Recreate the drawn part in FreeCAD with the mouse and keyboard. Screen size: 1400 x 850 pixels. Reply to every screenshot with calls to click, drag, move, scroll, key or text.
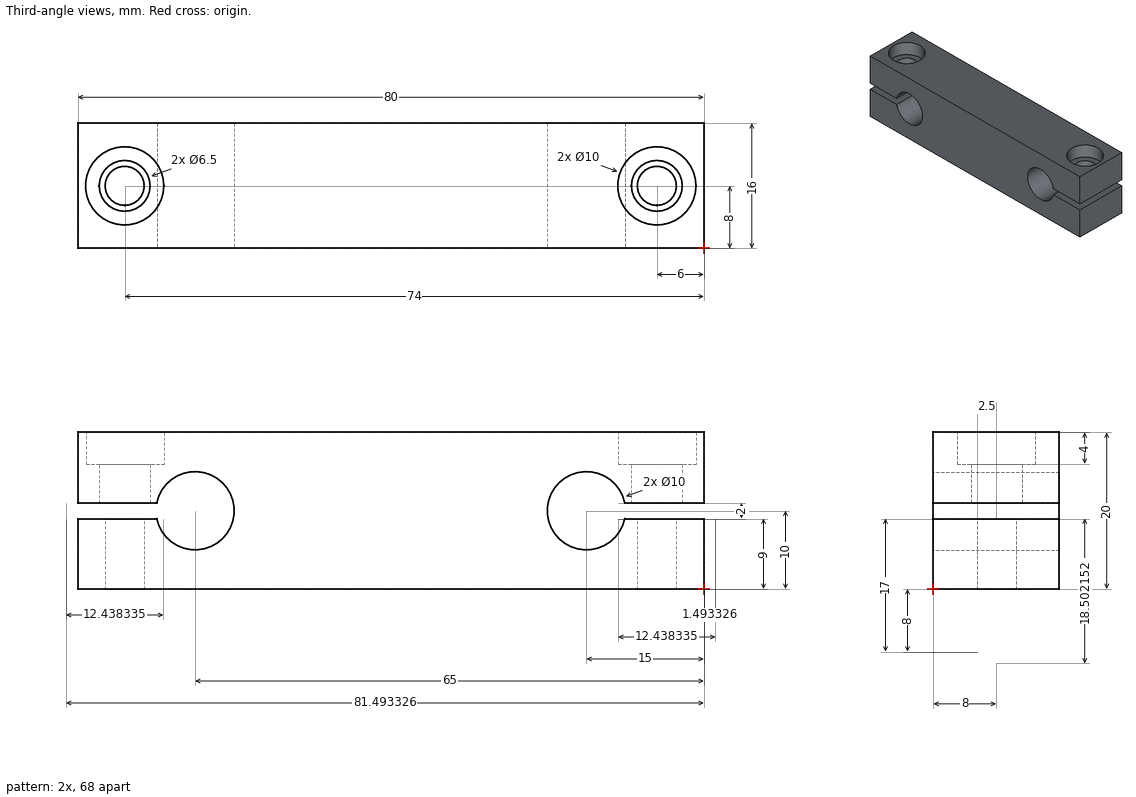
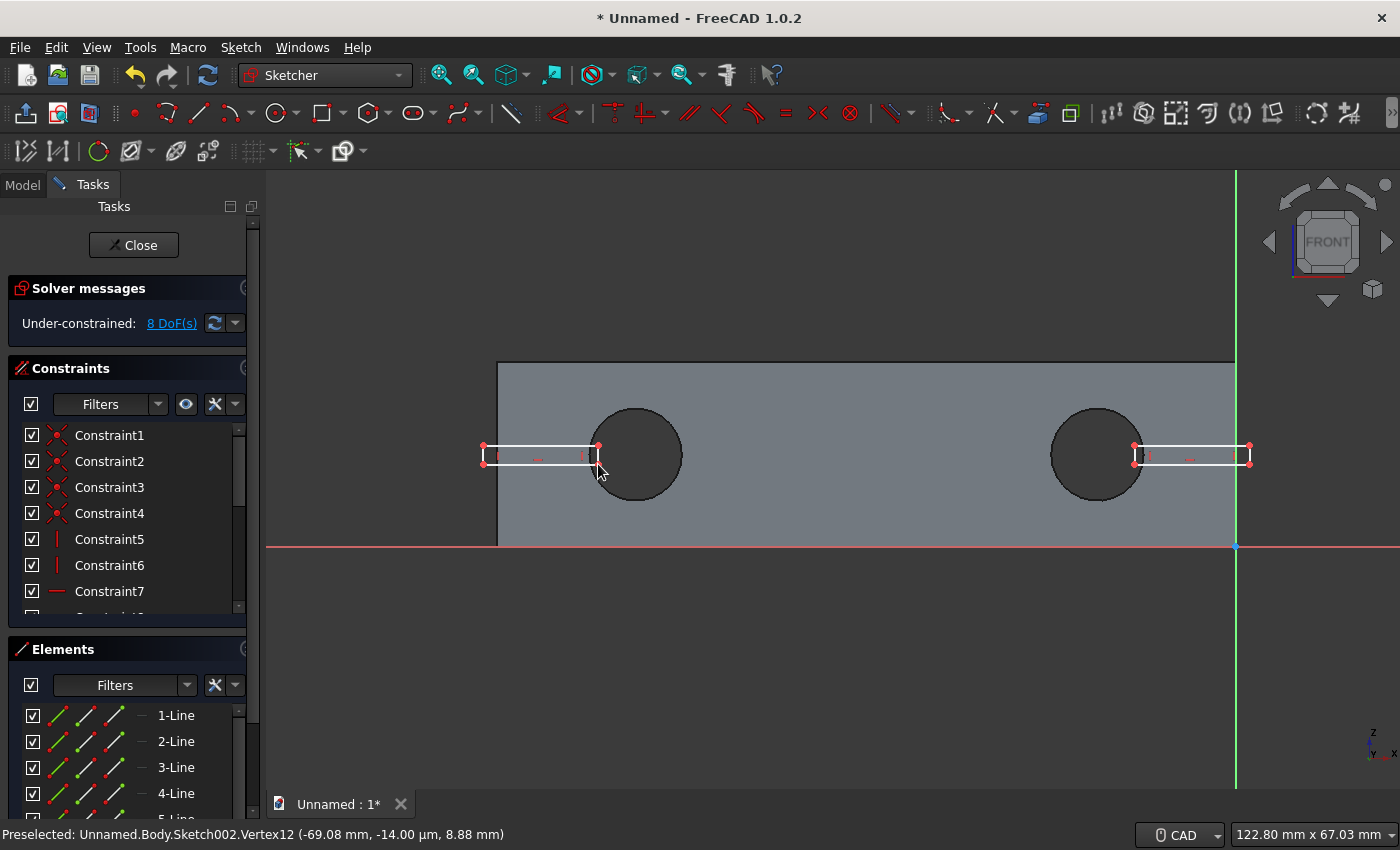
click(558, 114)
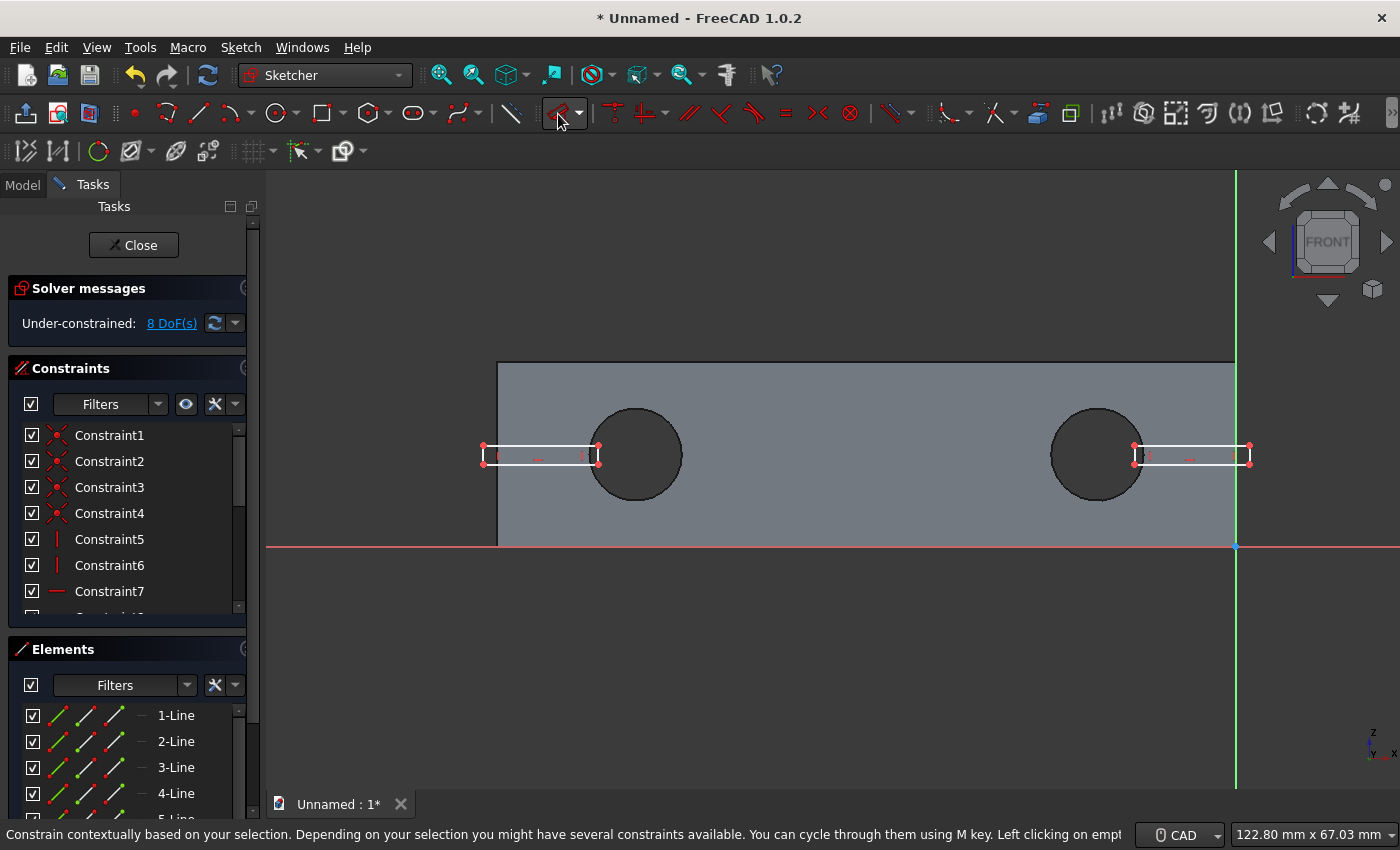
scroll(1135, 455, up, 4)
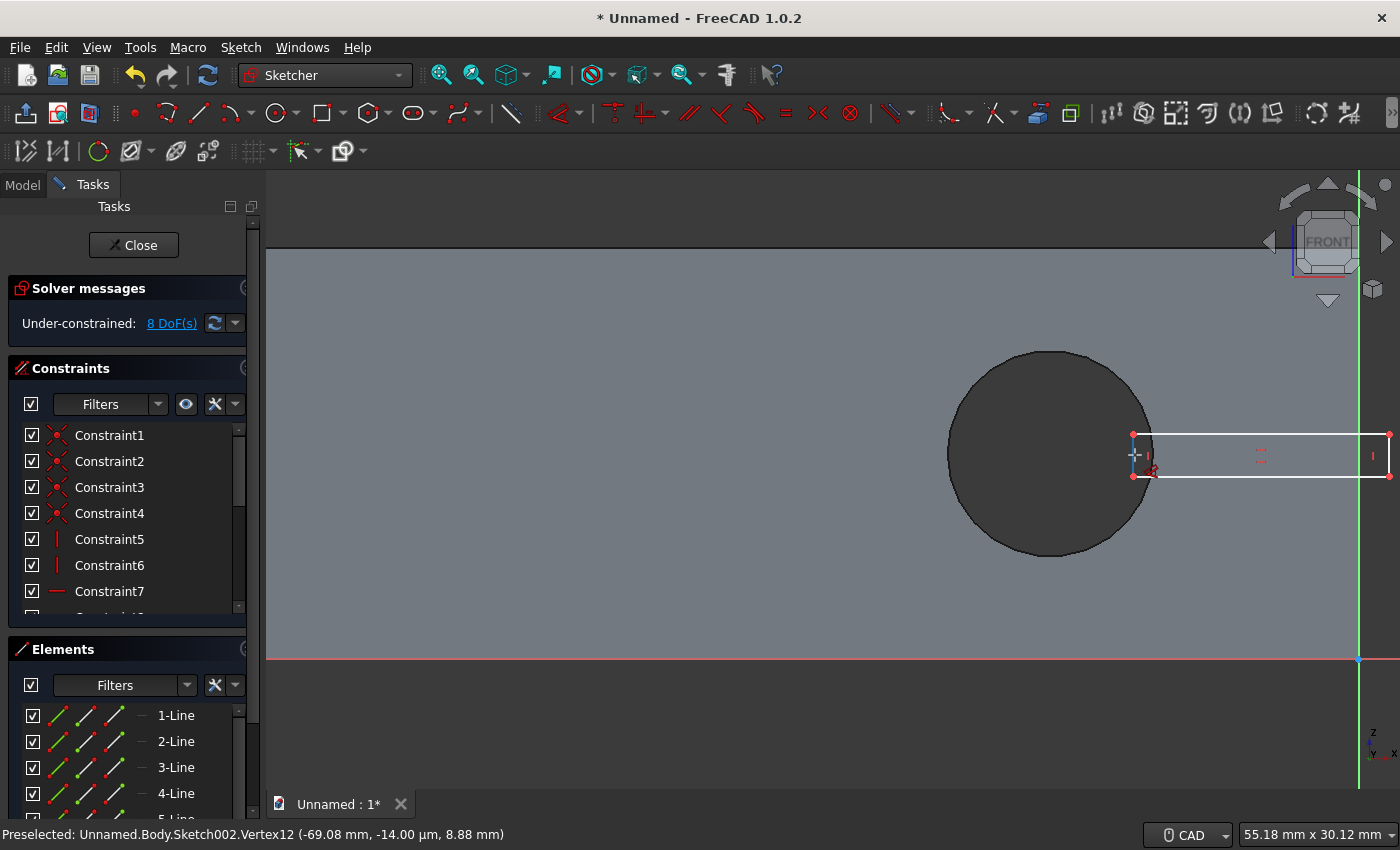
click(1133, 456)
click(1167, 456)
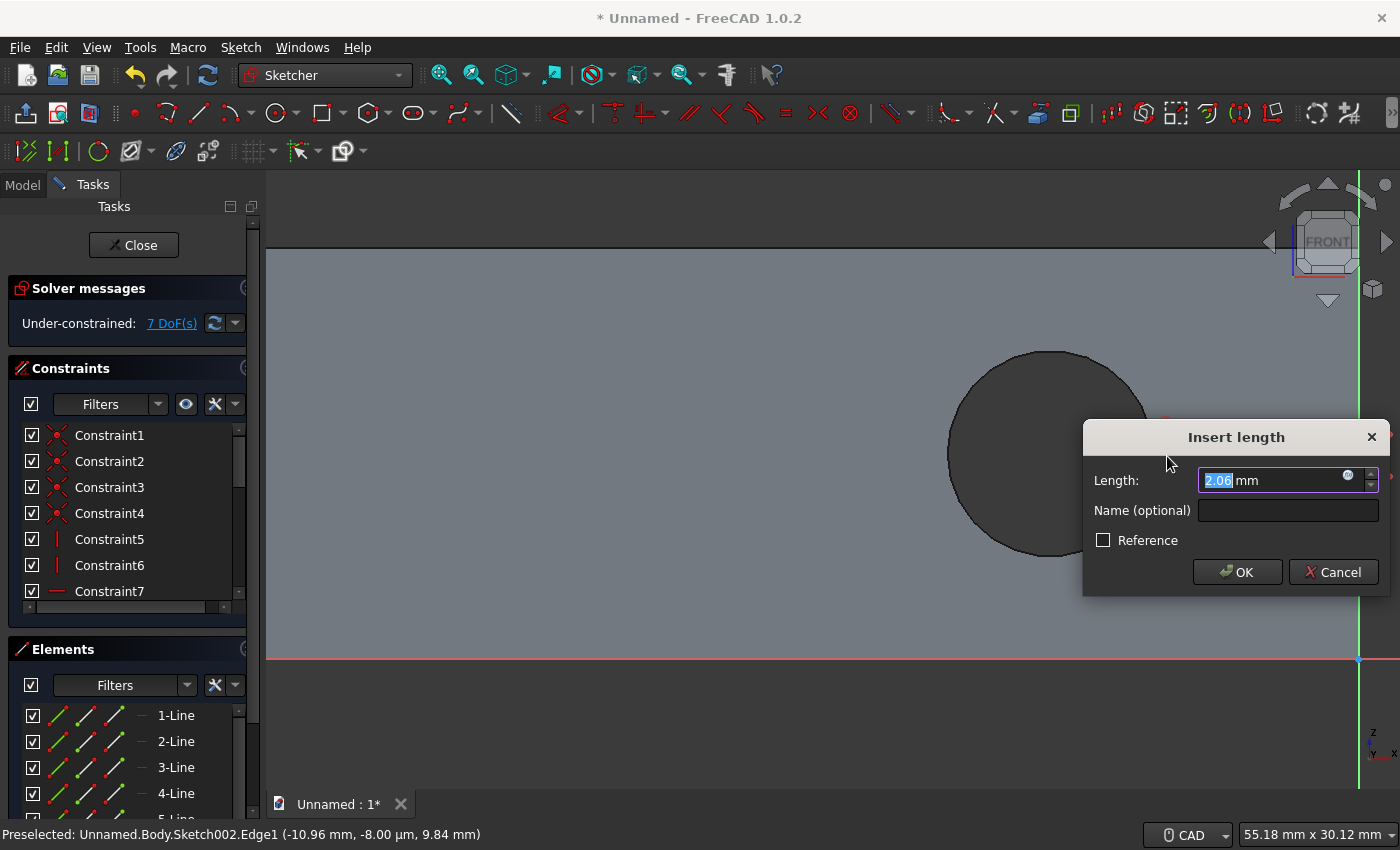
text(2)
key(Return)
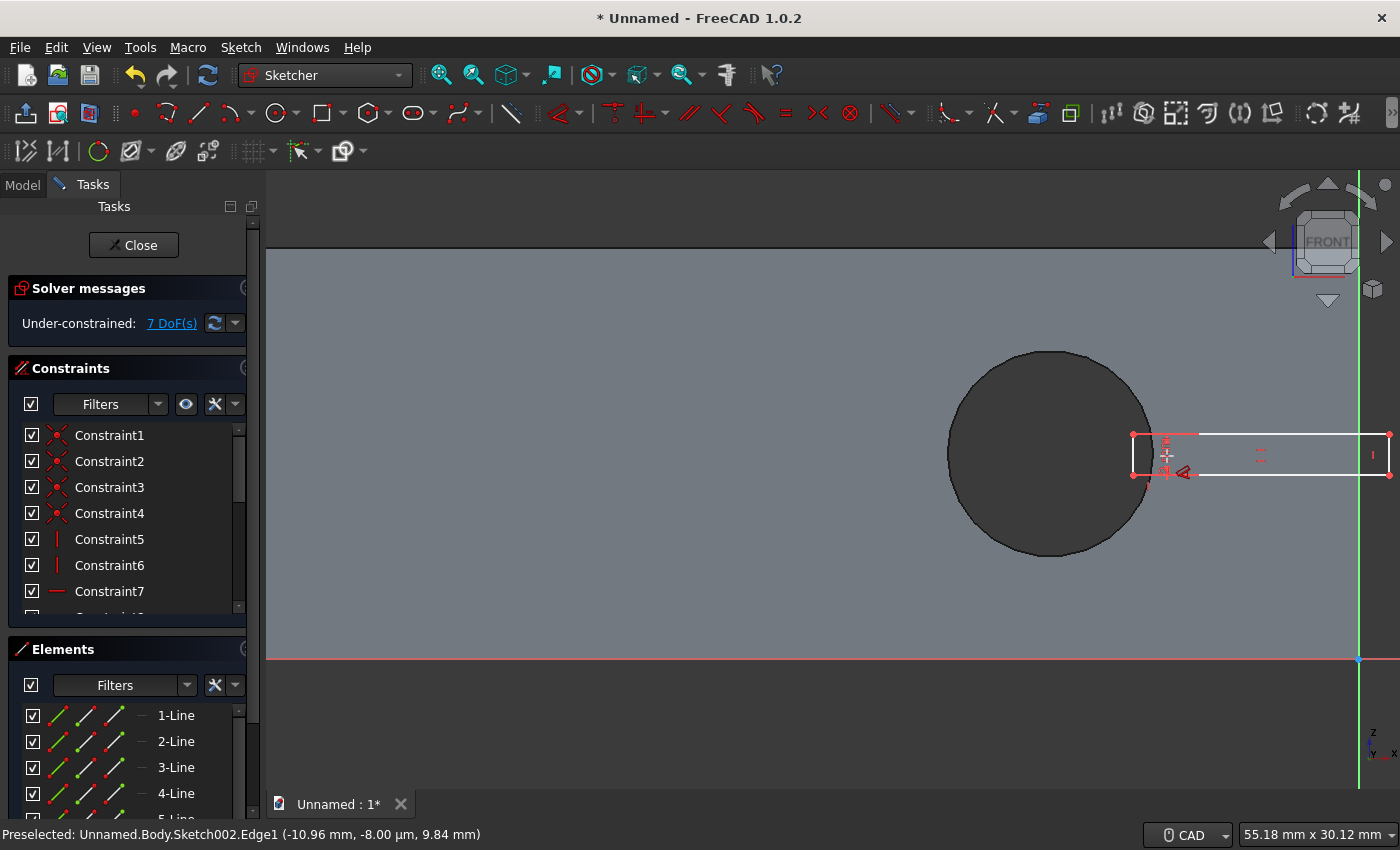
scroll(897, 441, down, 5)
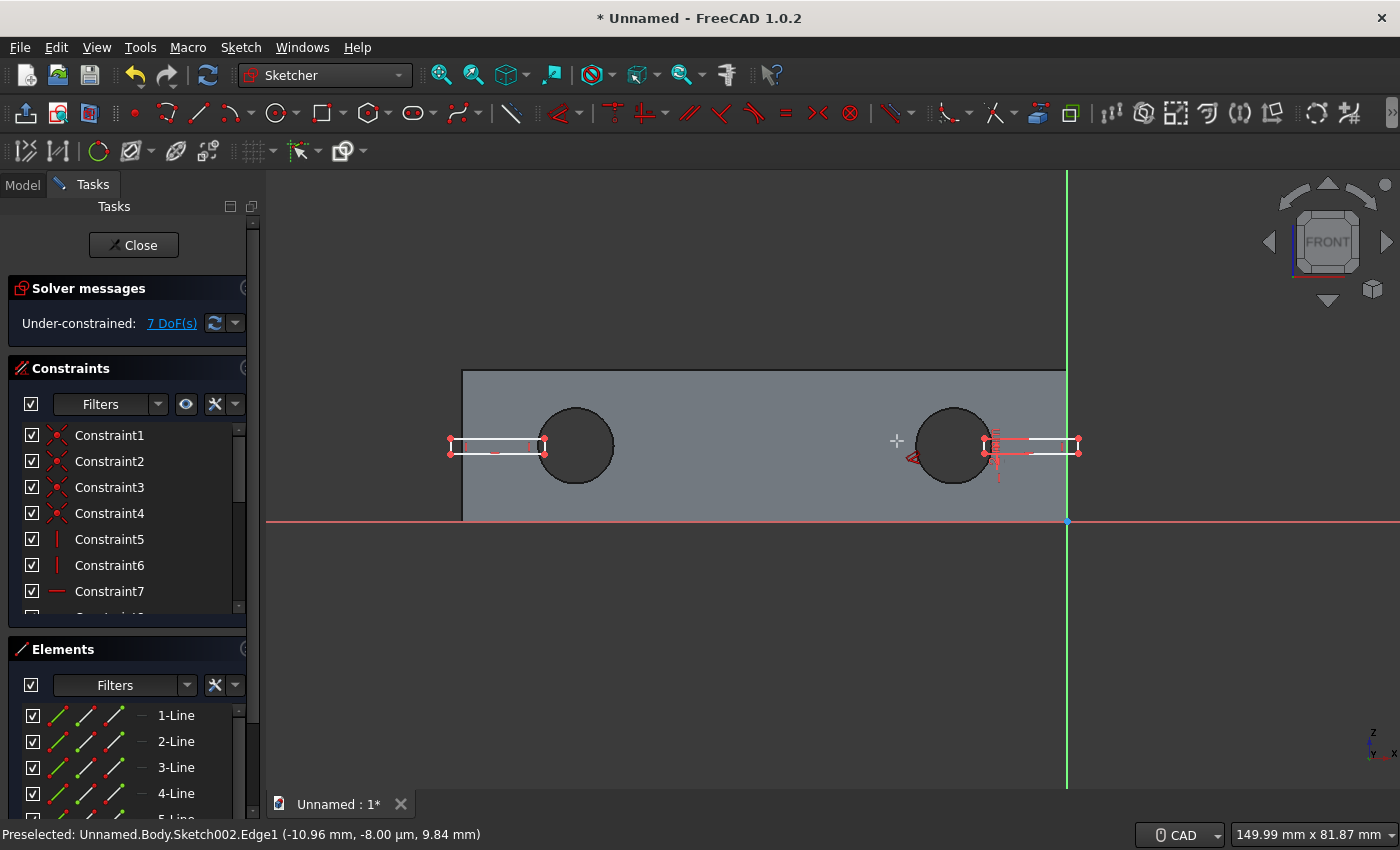
scroll(451, 444, up, 6)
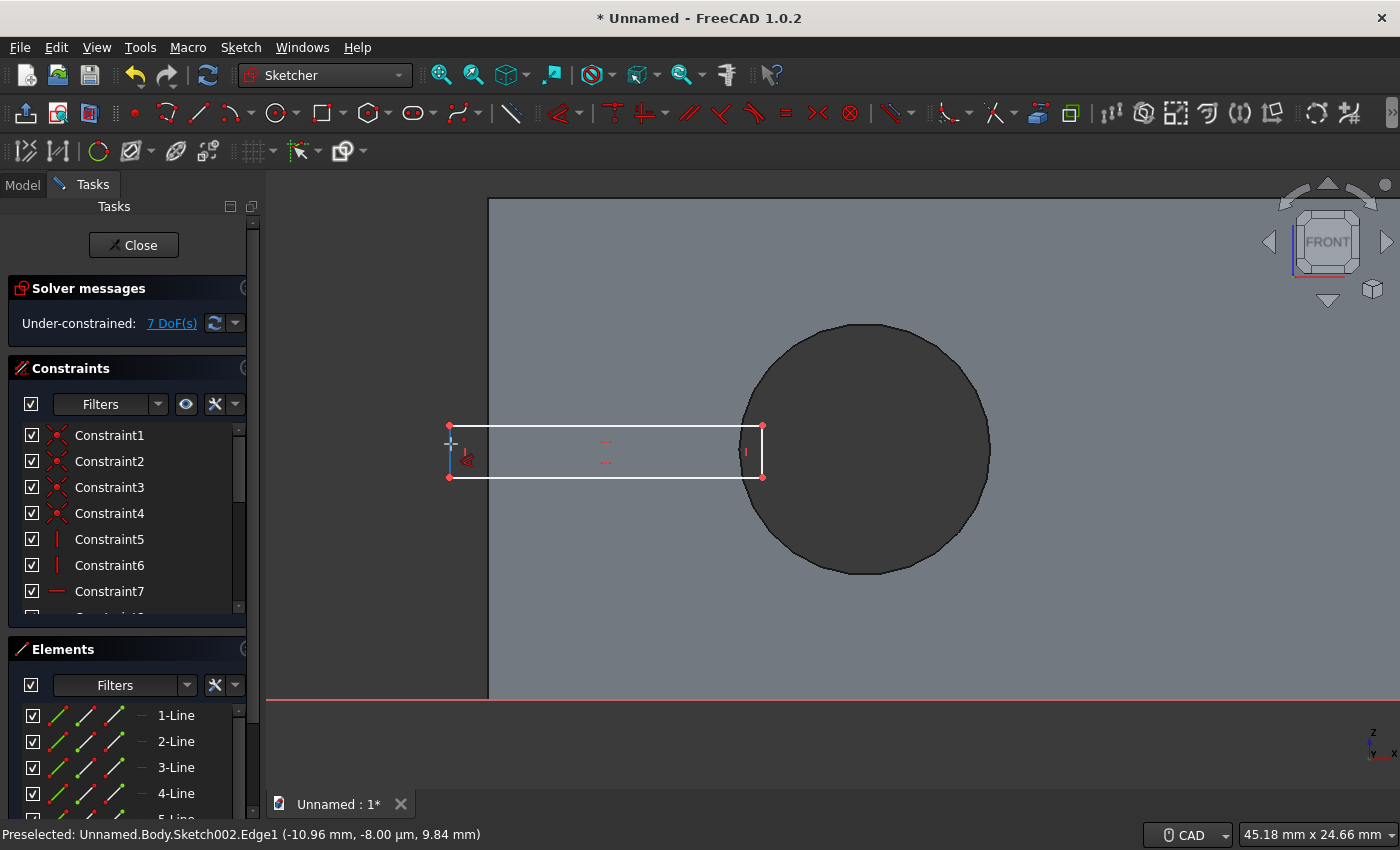
click(450, 441)
click(416, 452)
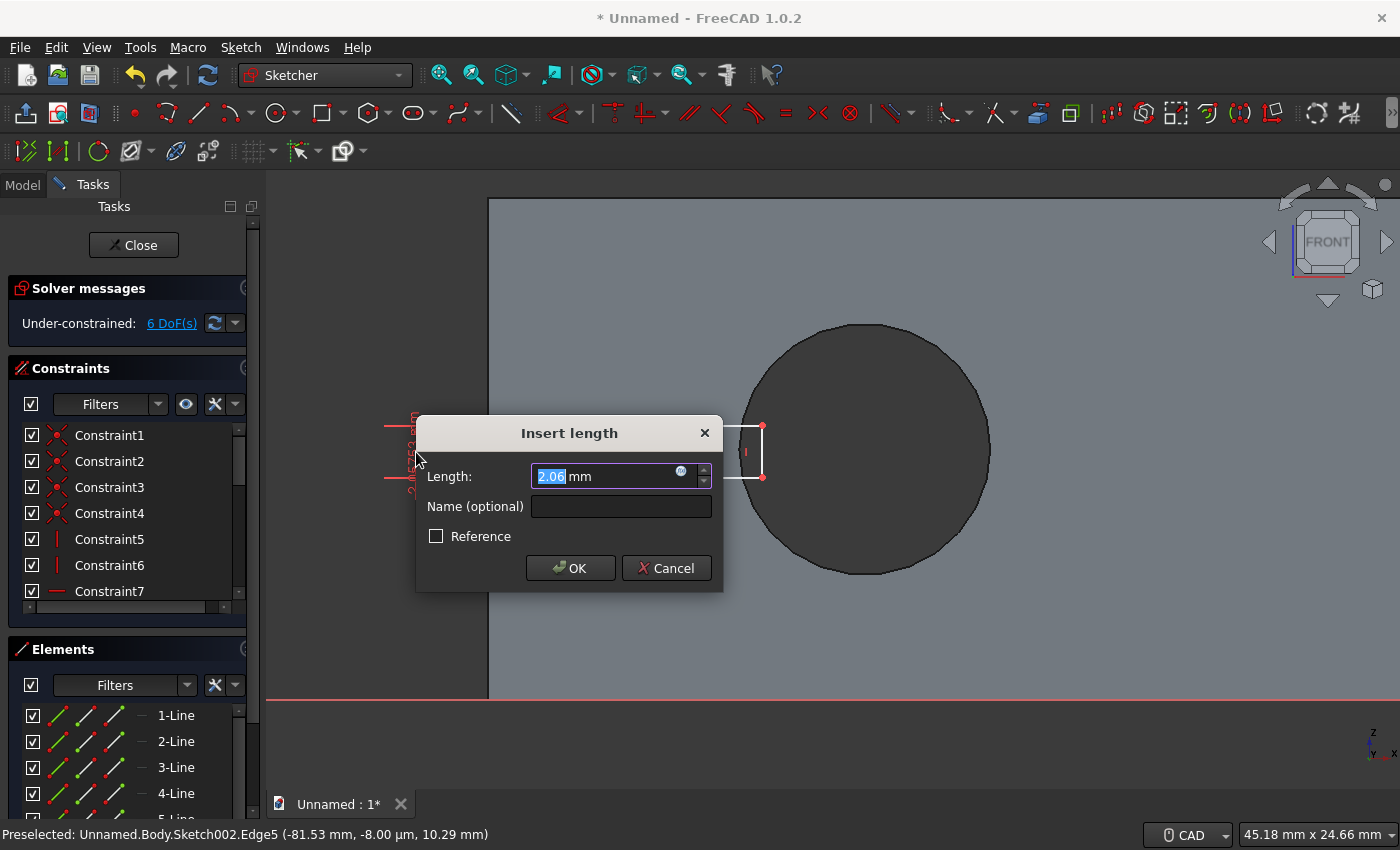
text(2)
key(Return)